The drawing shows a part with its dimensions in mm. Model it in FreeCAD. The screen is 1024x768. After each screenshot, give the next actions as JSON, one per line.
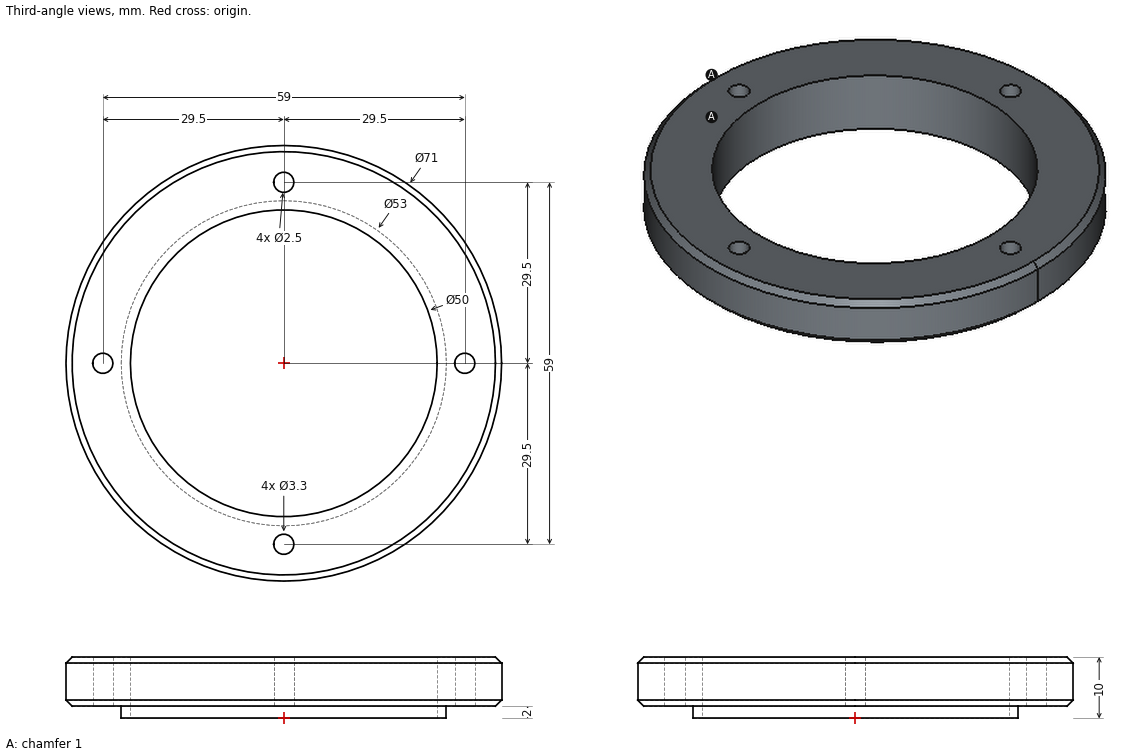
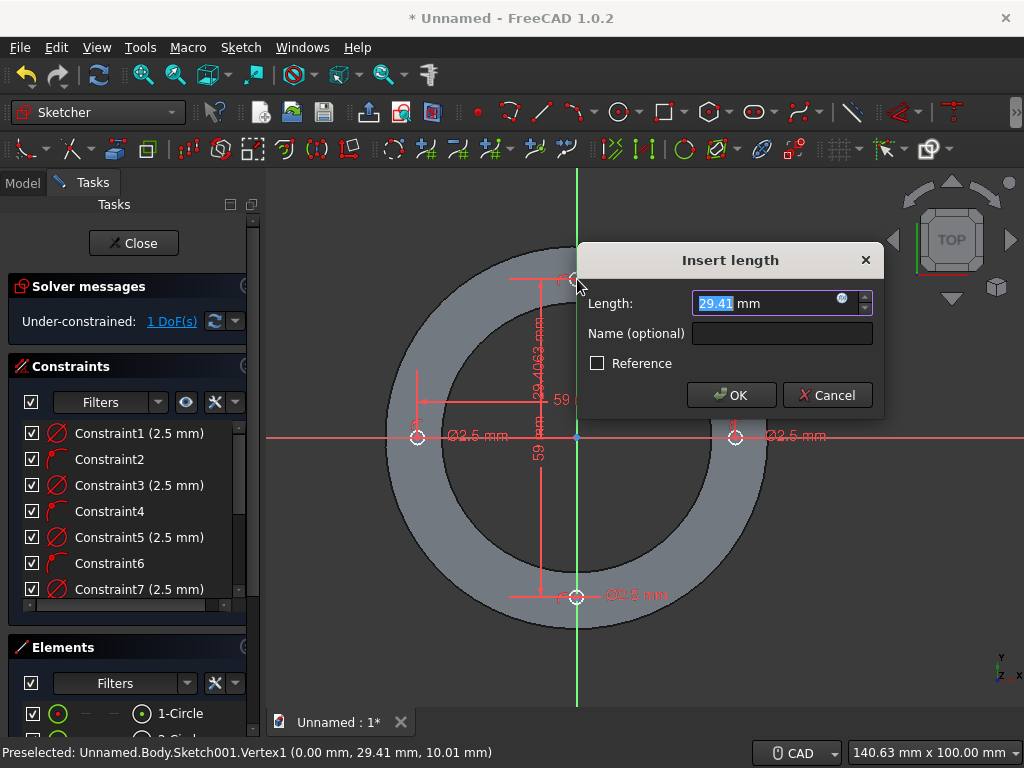
{"action": "type", "text": "29.5"}
{"action": "key", "text": "Return"}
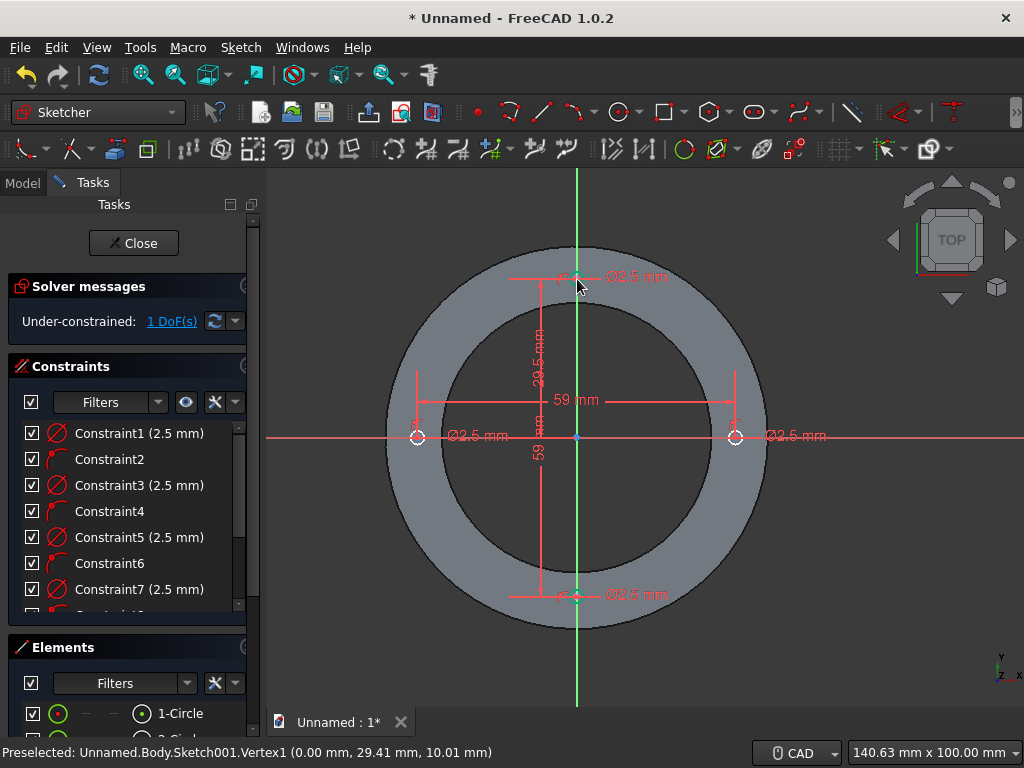
{"action": "left_click", "coordinate": [735, 438]}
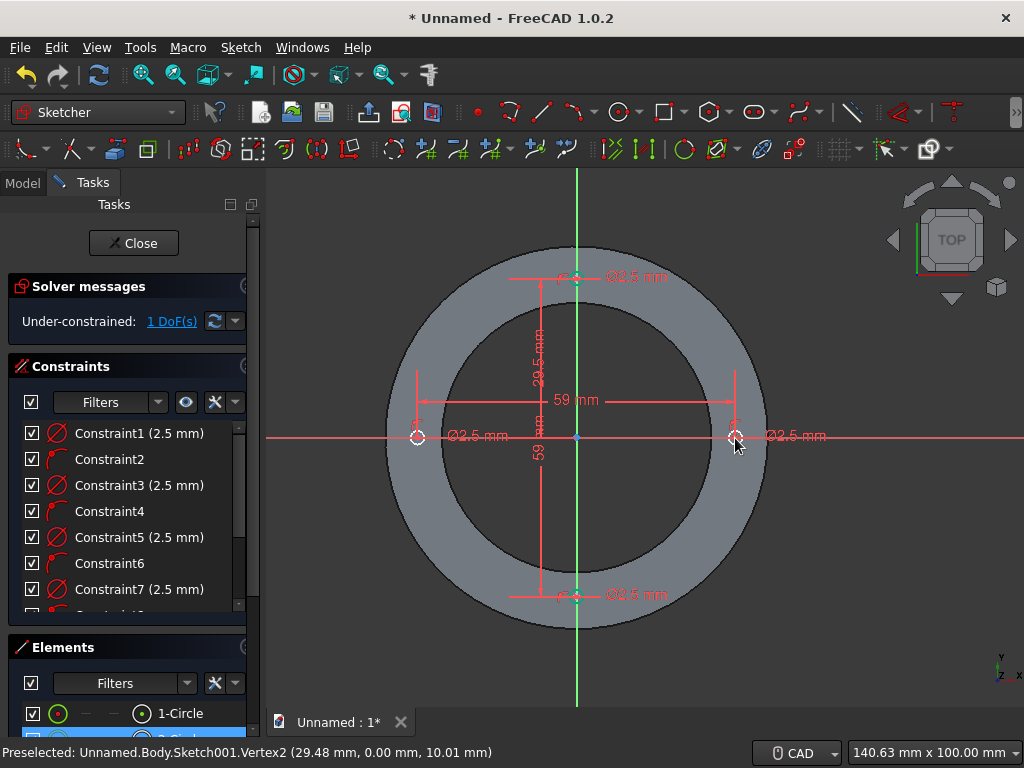
{"action": "key", "text": "l"}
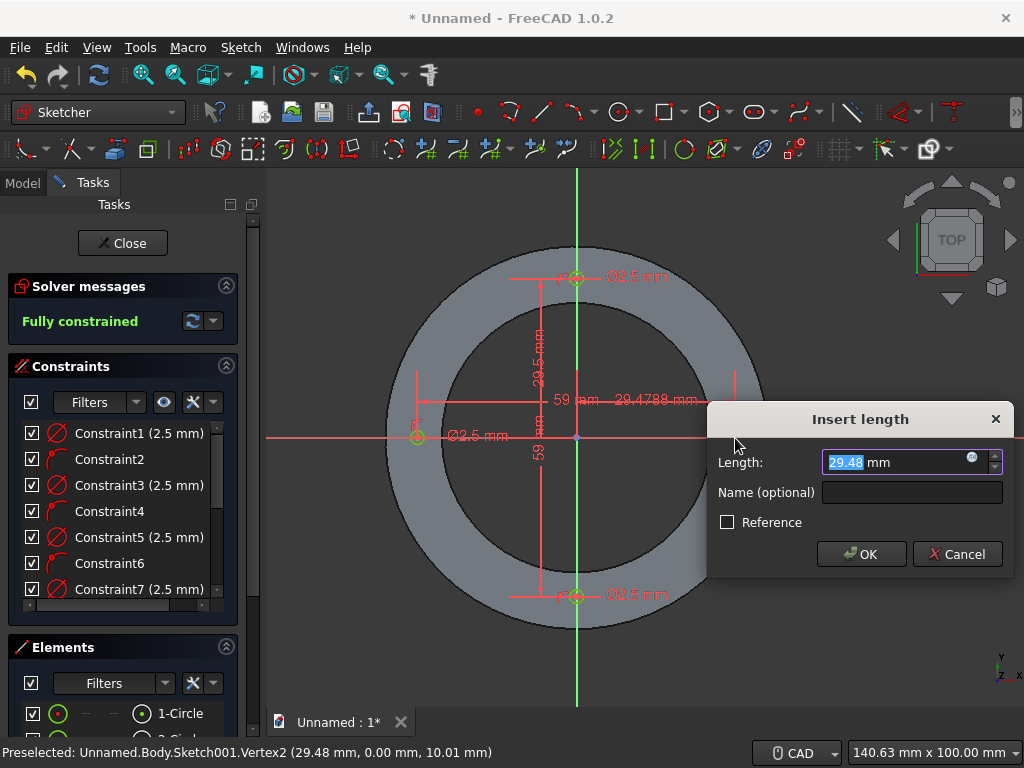
{"action": "type", "text": "29.5"}
{"action": "key", "text": "Return"}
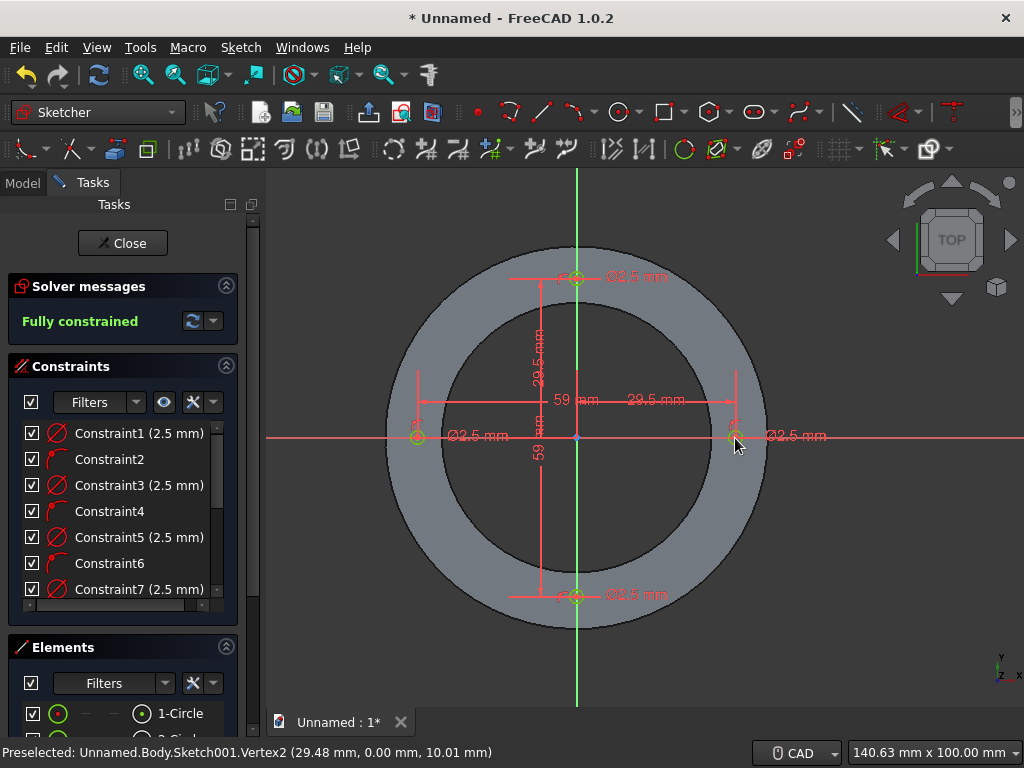
{"action": "left_click", "coordinate": [123, 243]}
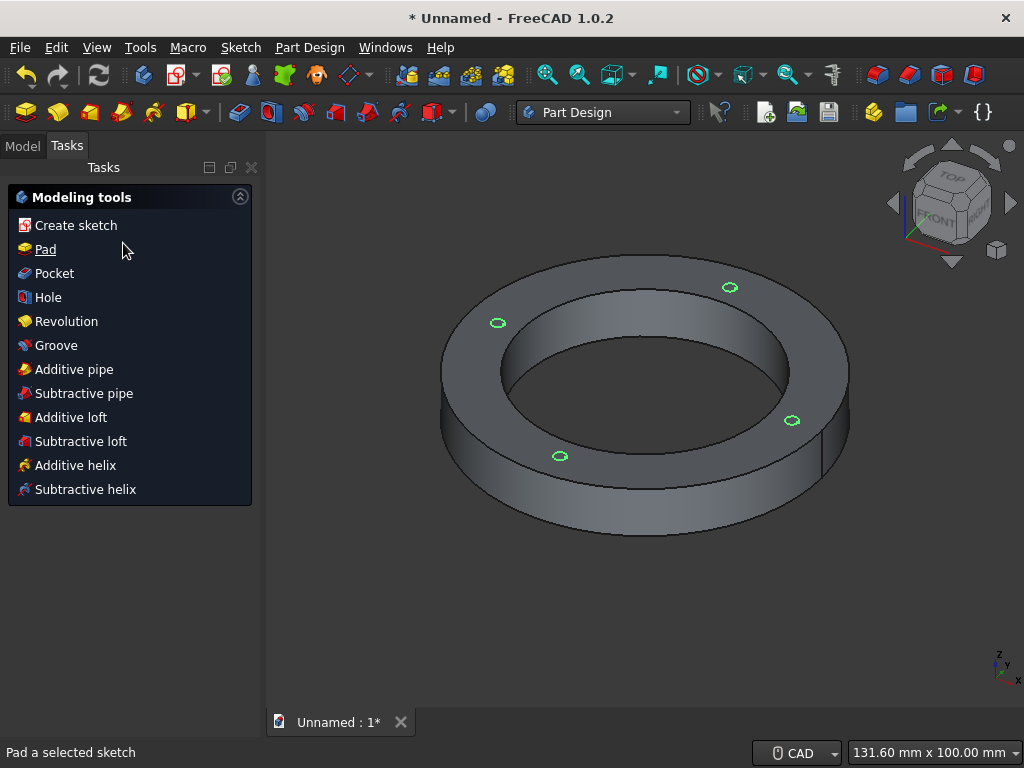
{"action": "left_click", "coordinate": [240, 112]}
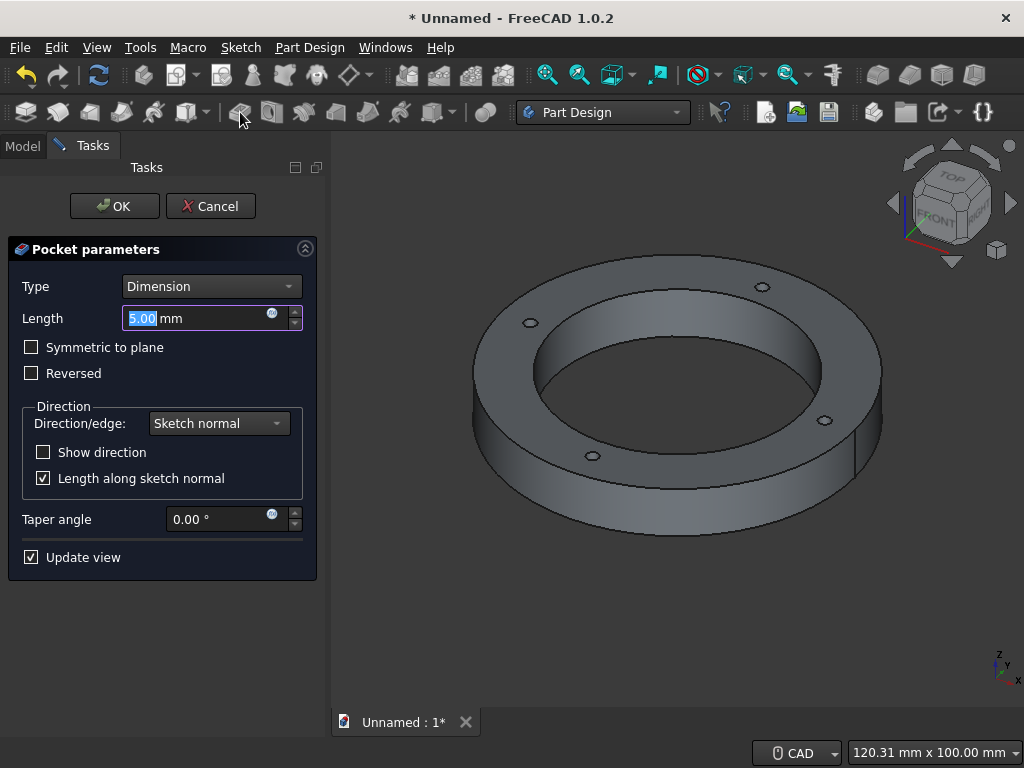
{"action": "left_click", "coordinate": [212, 286]}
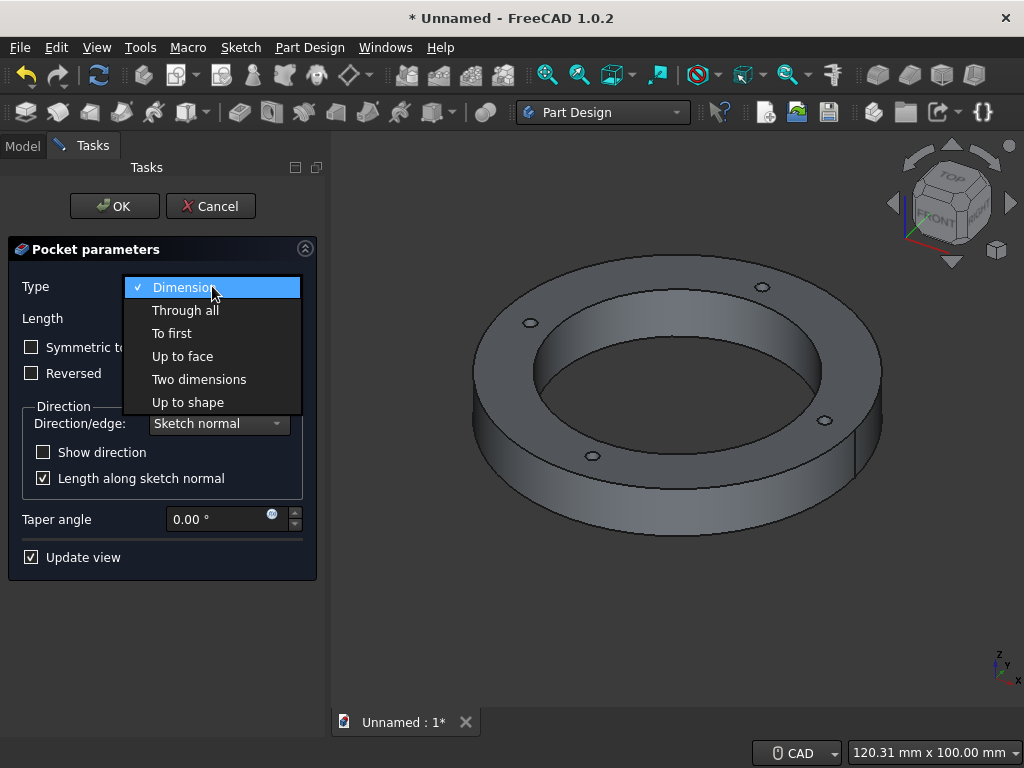
{"action": "left_click", "coordinate": [212, 310]}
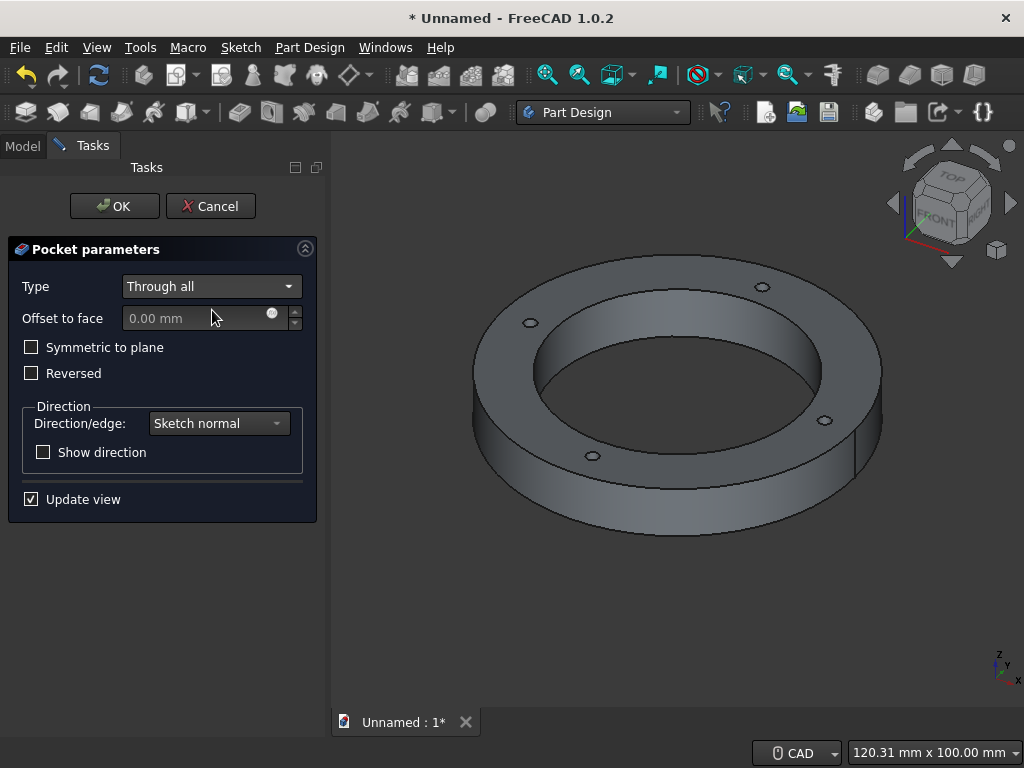
{"action": "left_click", "coordinate": [115, 206]}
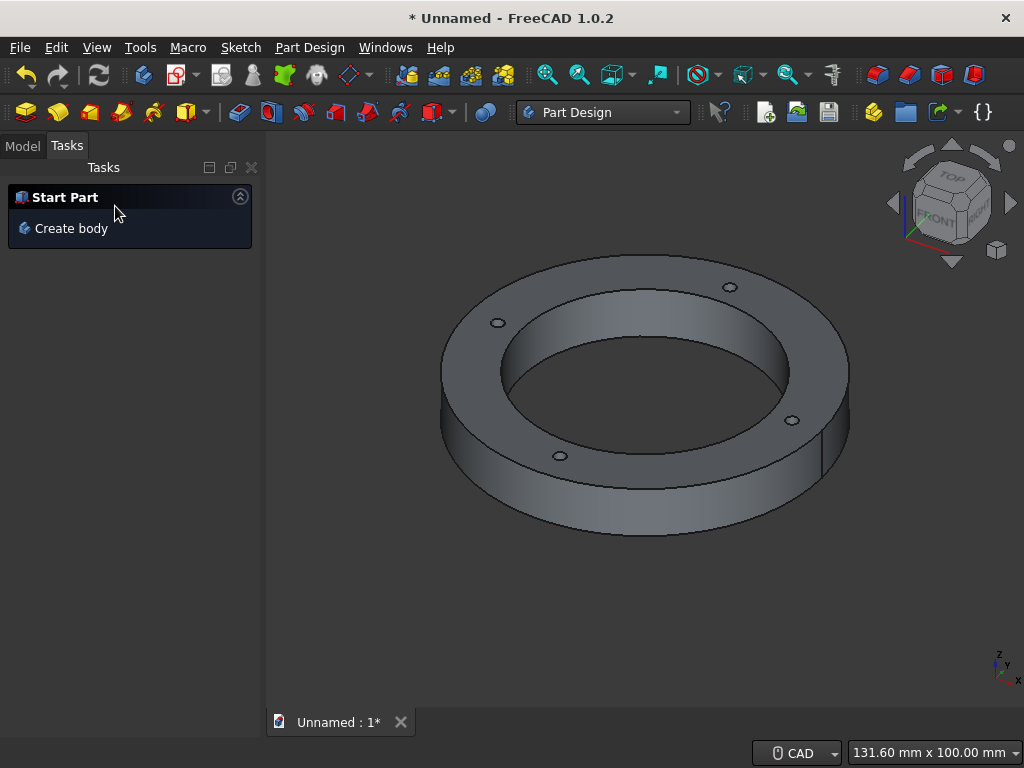
{"action": "key", "text": "5"}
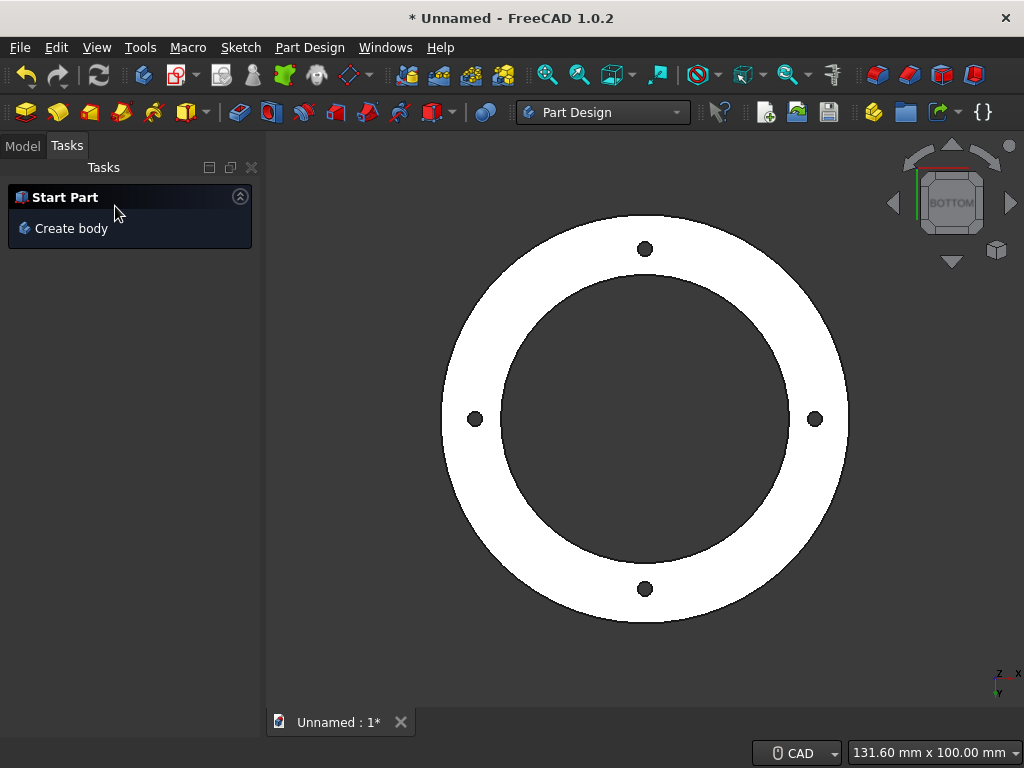
{"action": "left_click", "coordinate": [762, 535]}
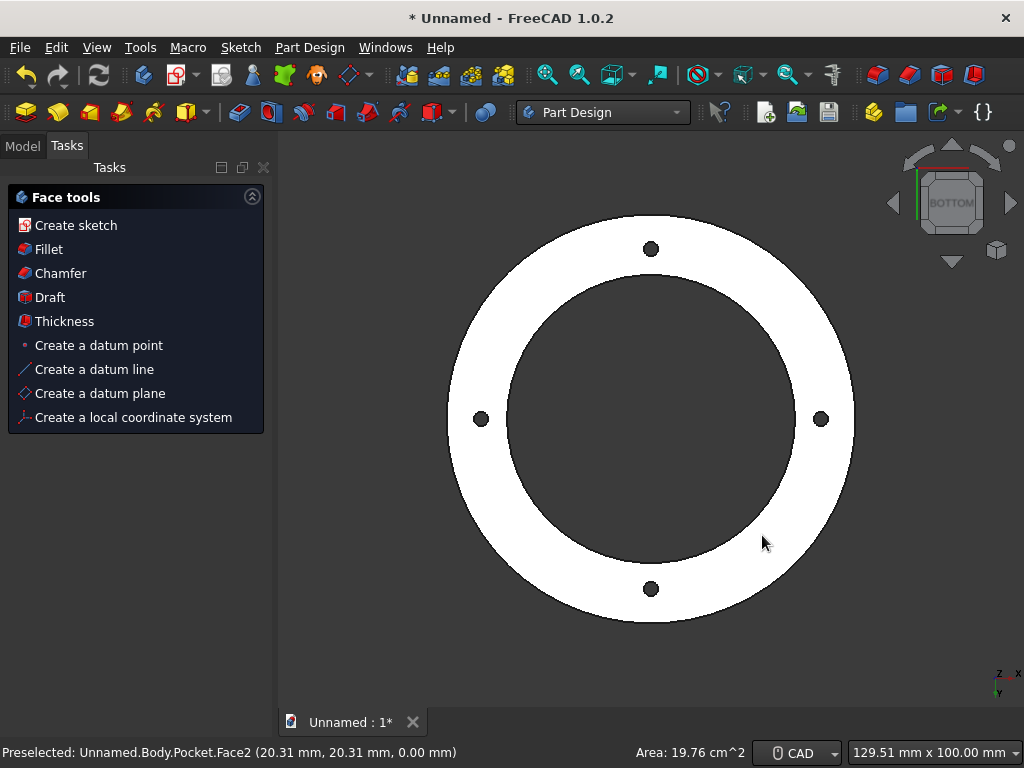
{"action": "left_click", "coordinate": [176, 76]}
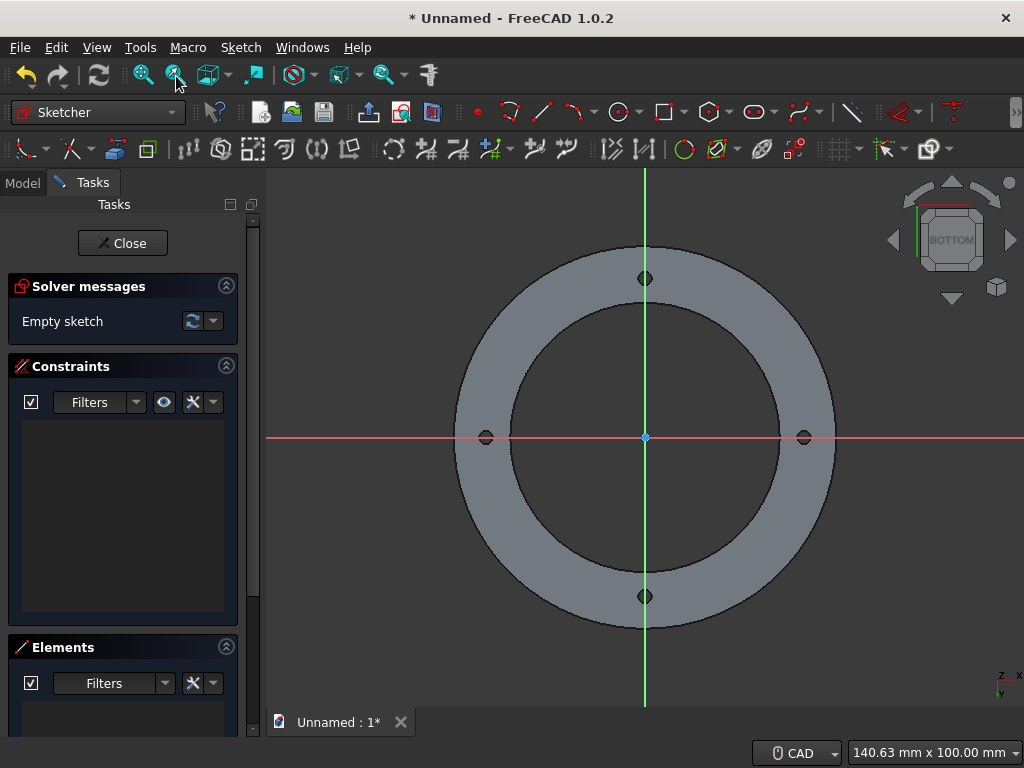
{"action": "scroll", "coordinate": [294, 437], "scroll_direction": "down", "scroll_amount": 1}